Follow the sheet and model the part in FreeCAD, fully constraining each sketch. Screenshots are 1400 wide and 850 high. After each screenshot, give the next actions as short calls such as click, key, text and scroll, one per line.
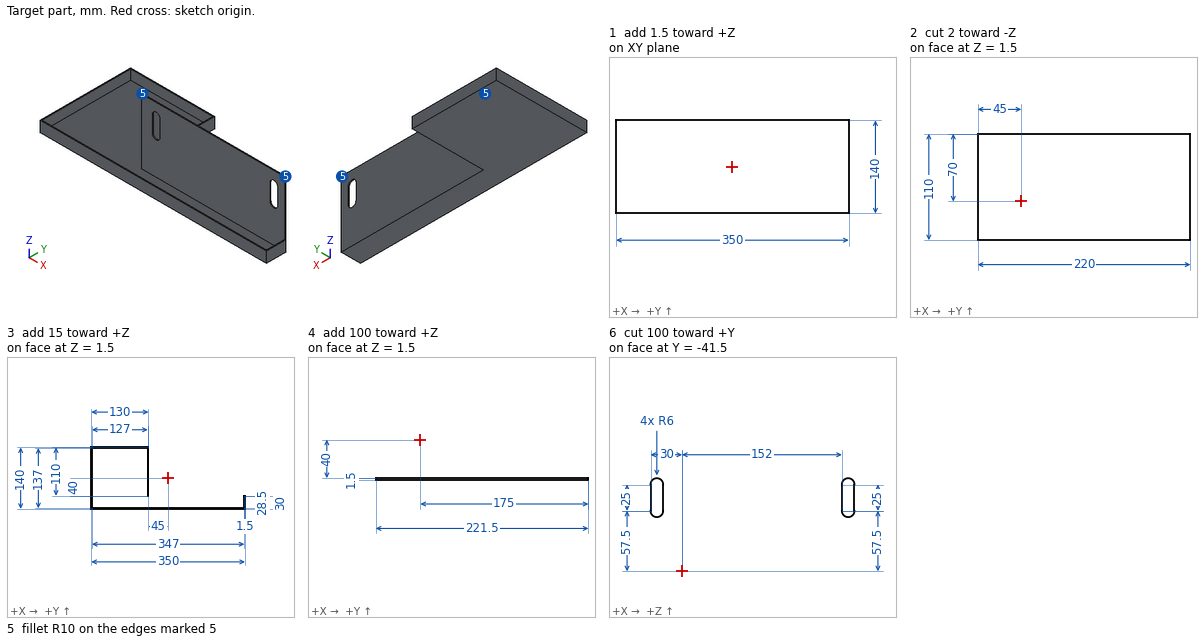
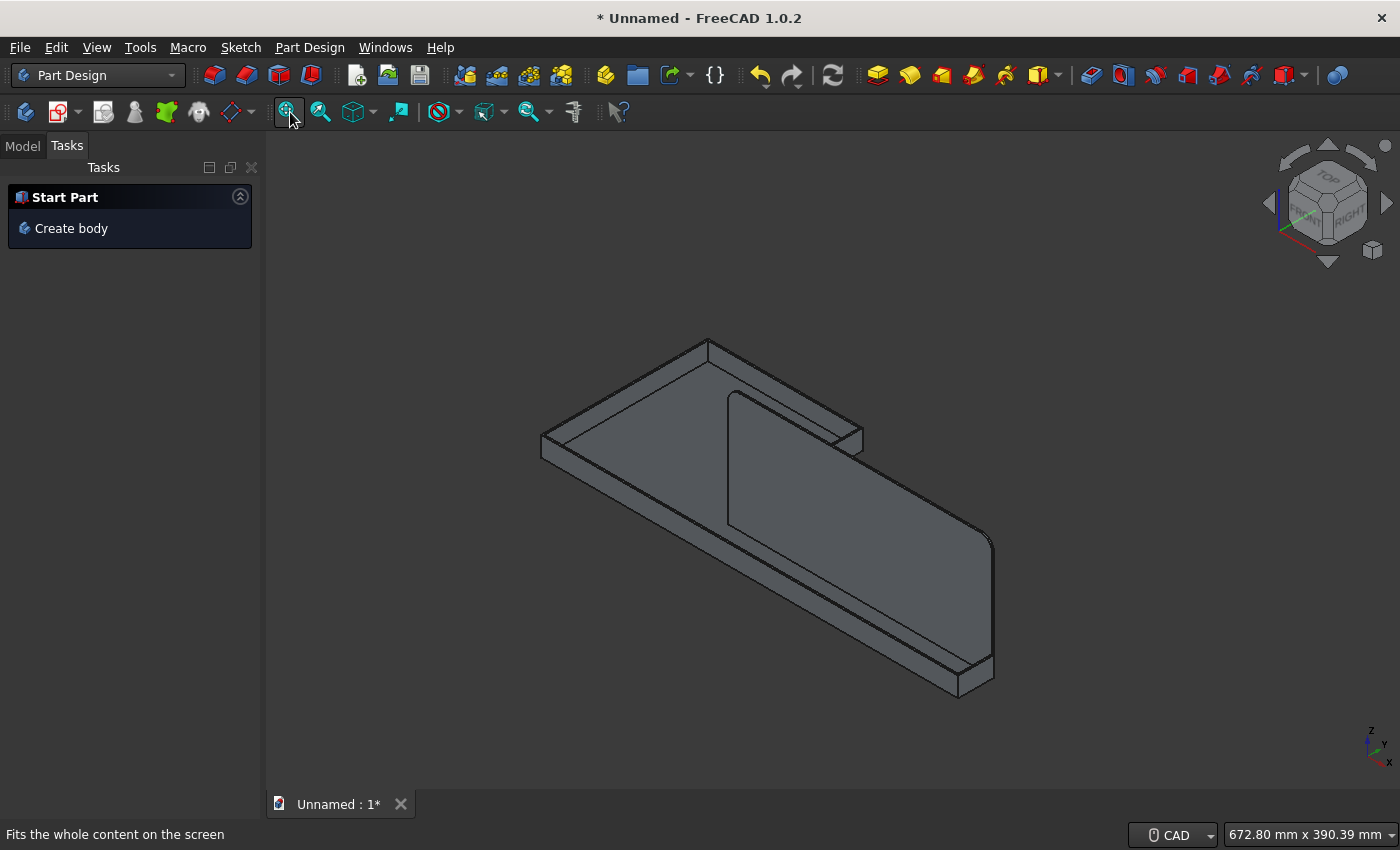
click(898, 553)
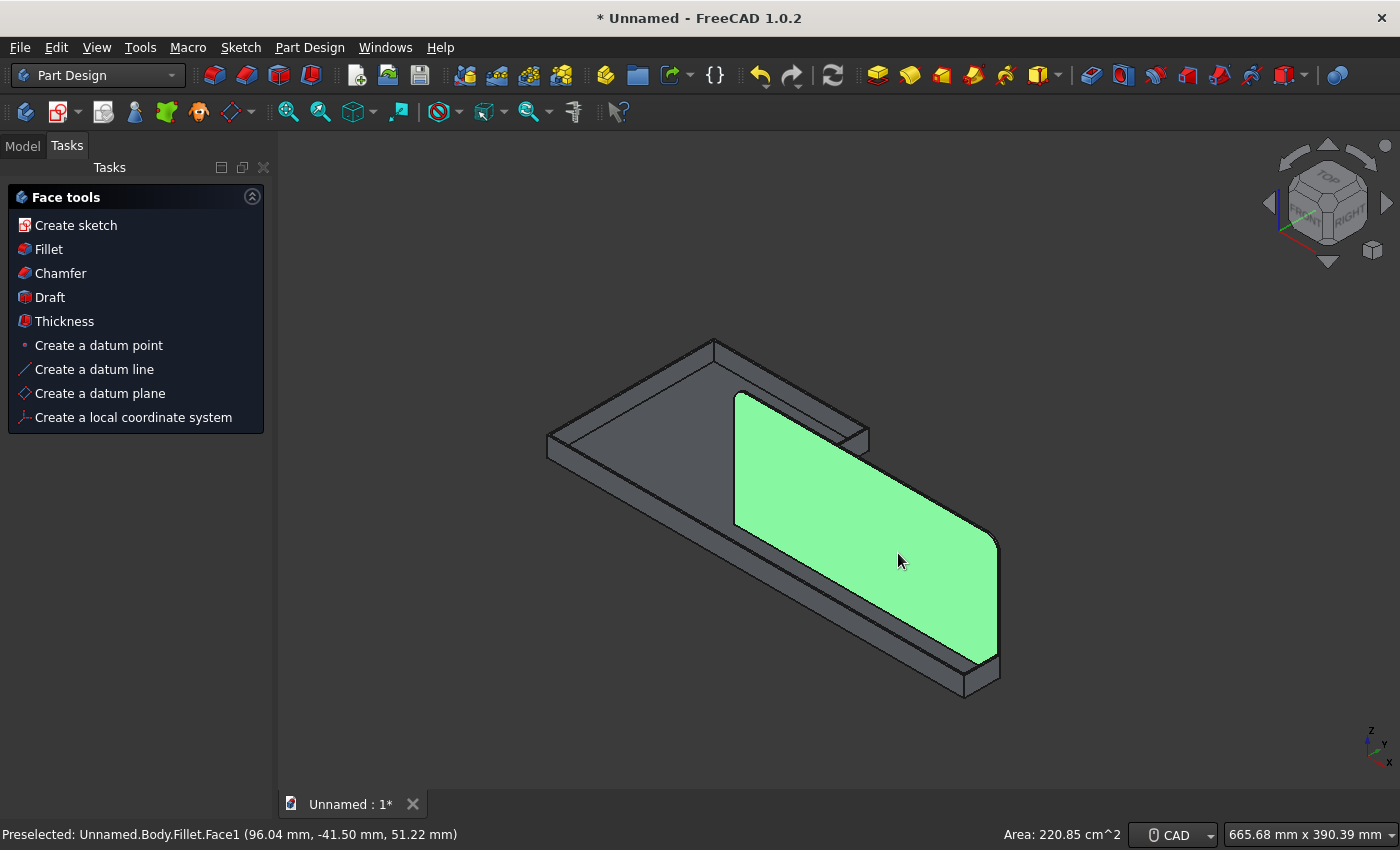
click(58, 112)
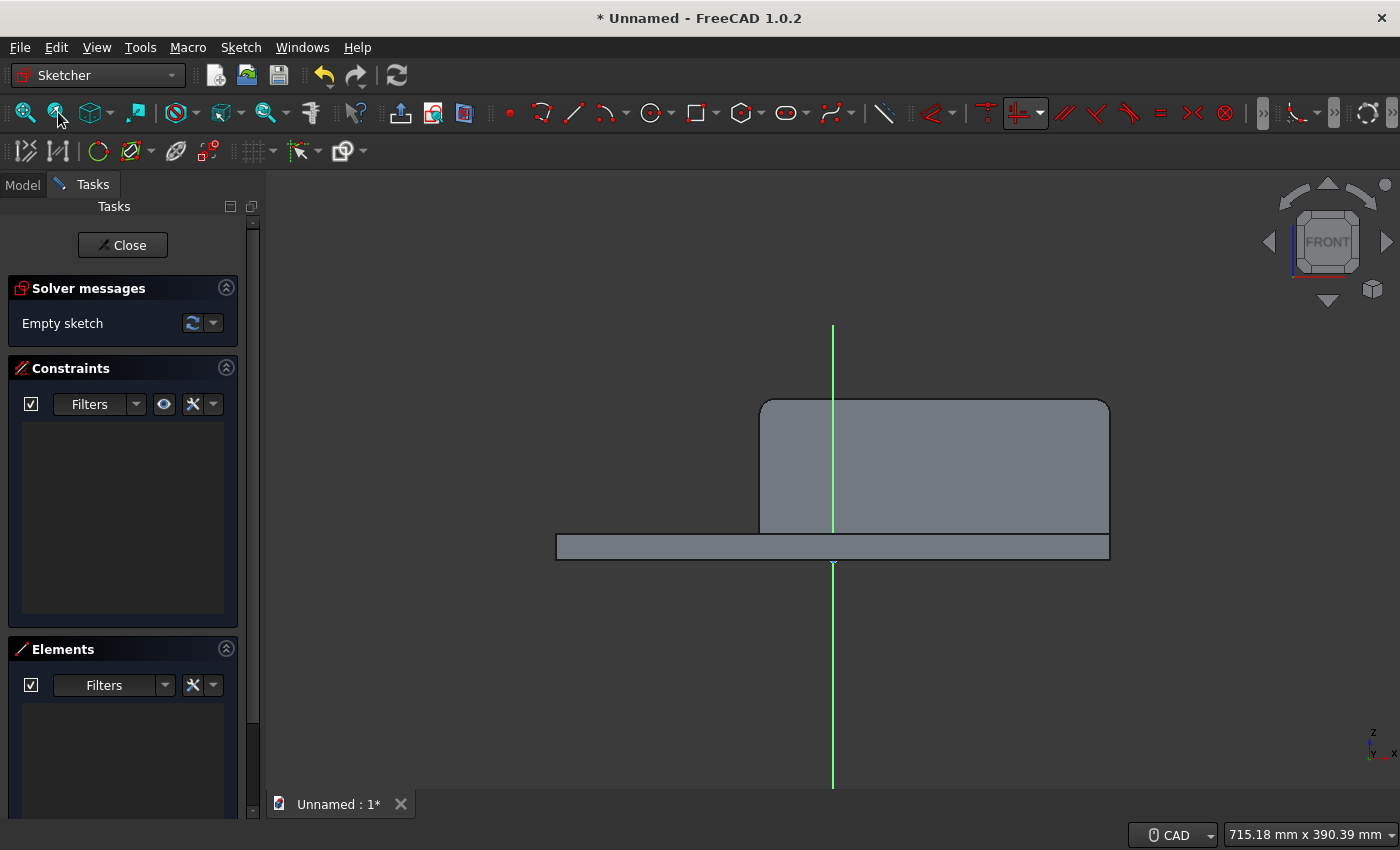
click(466, 114)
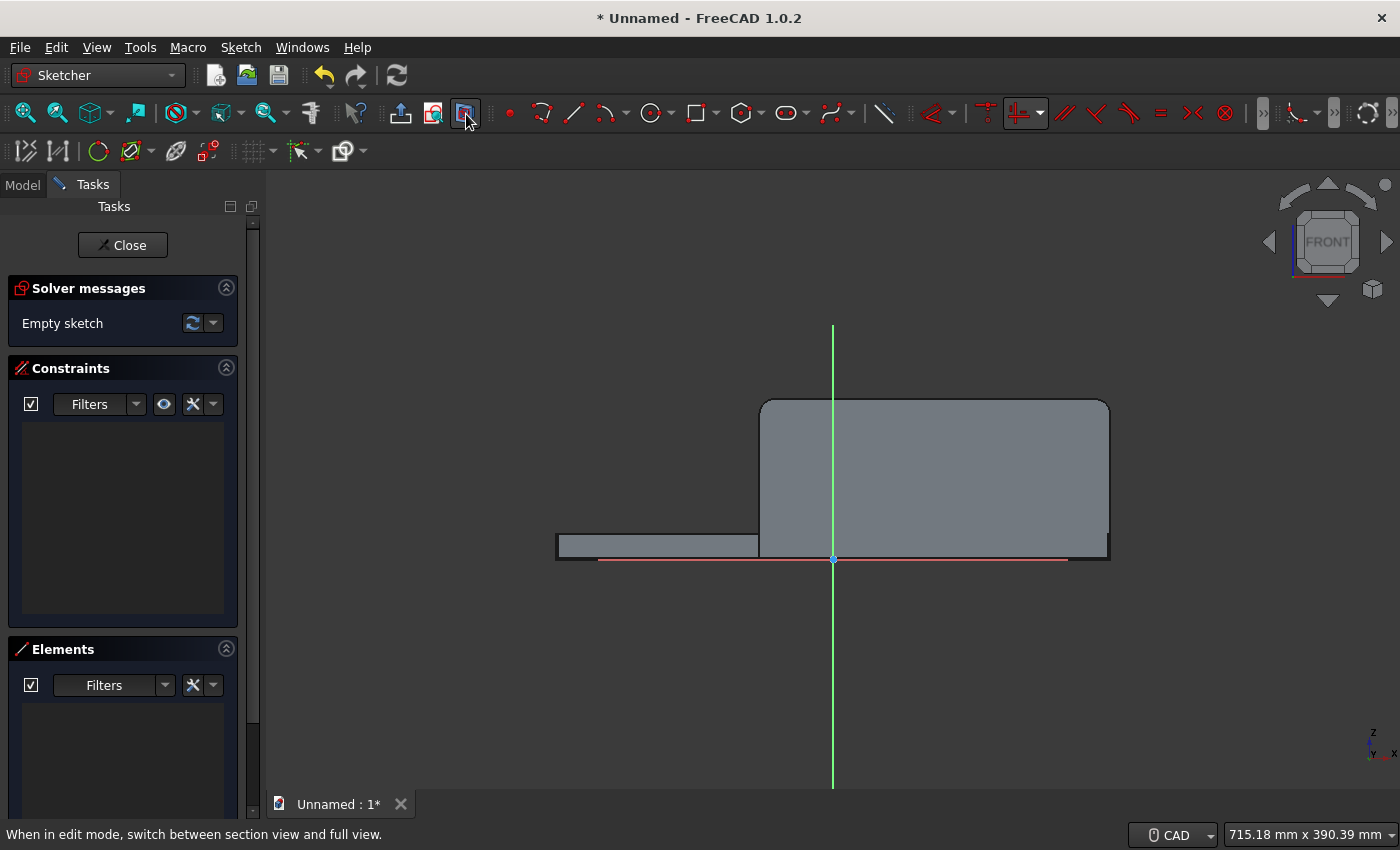
scroll(1082, 498, up, 4)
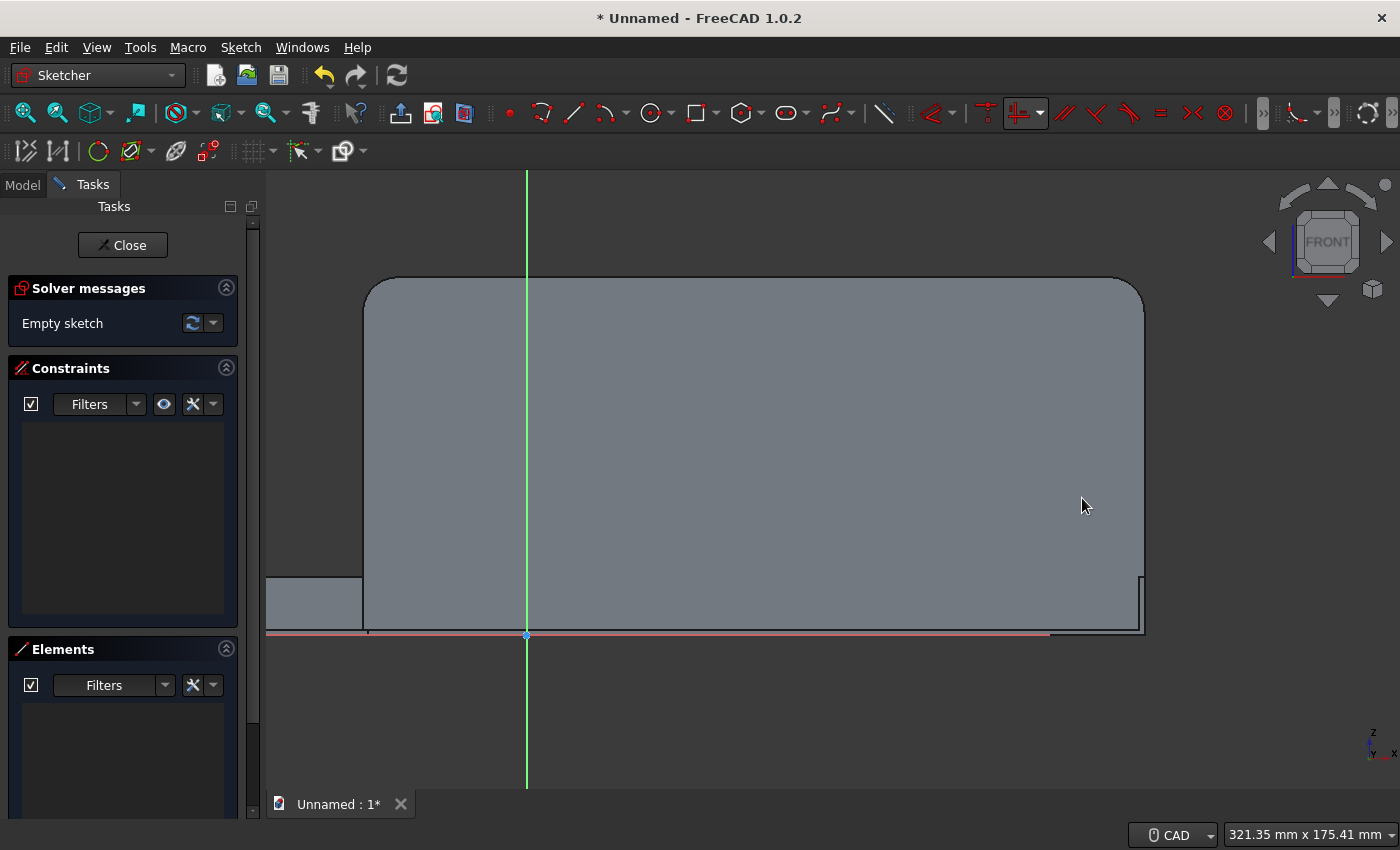
click(786, 114)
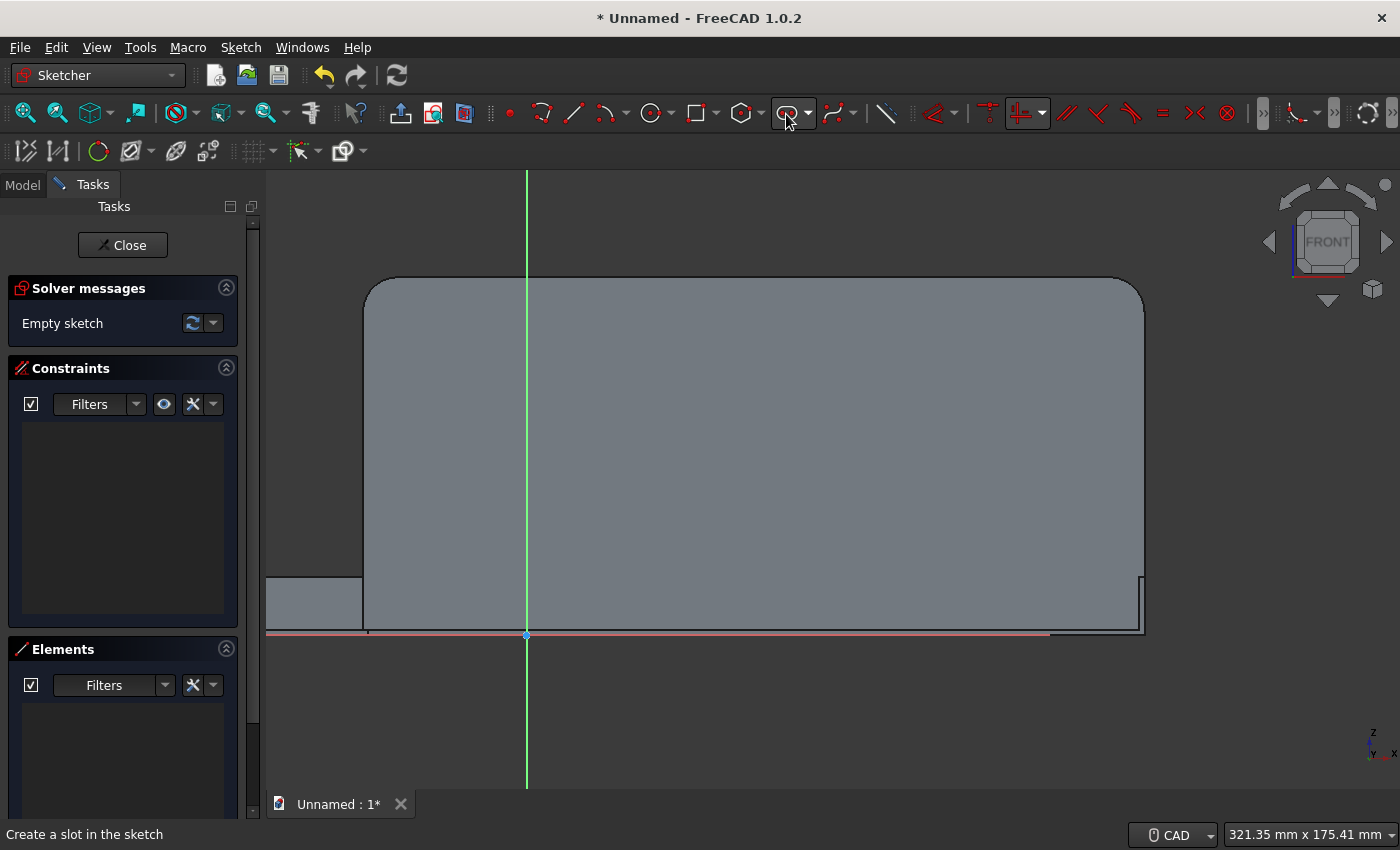
click(442, 432)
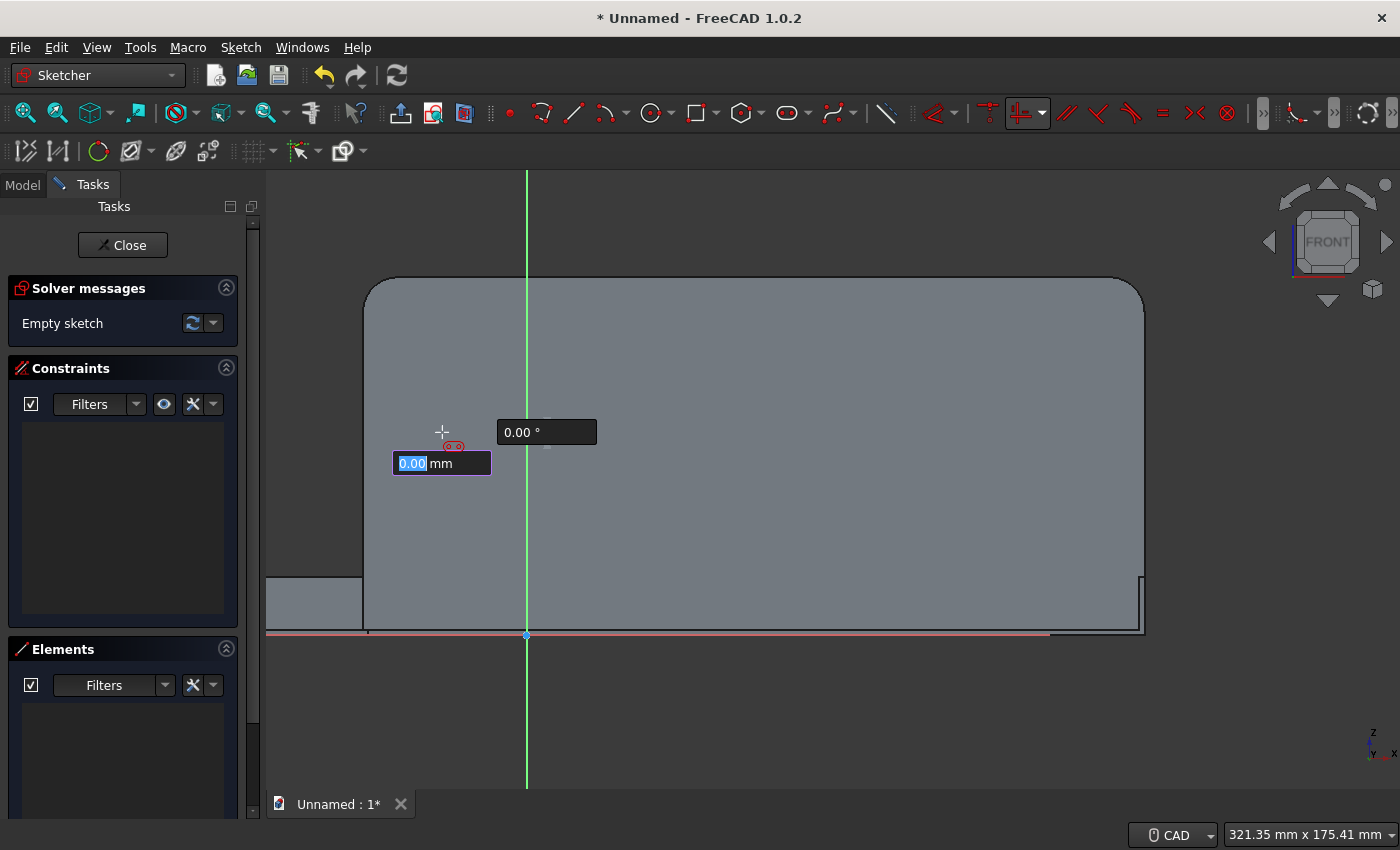
click(442, 344)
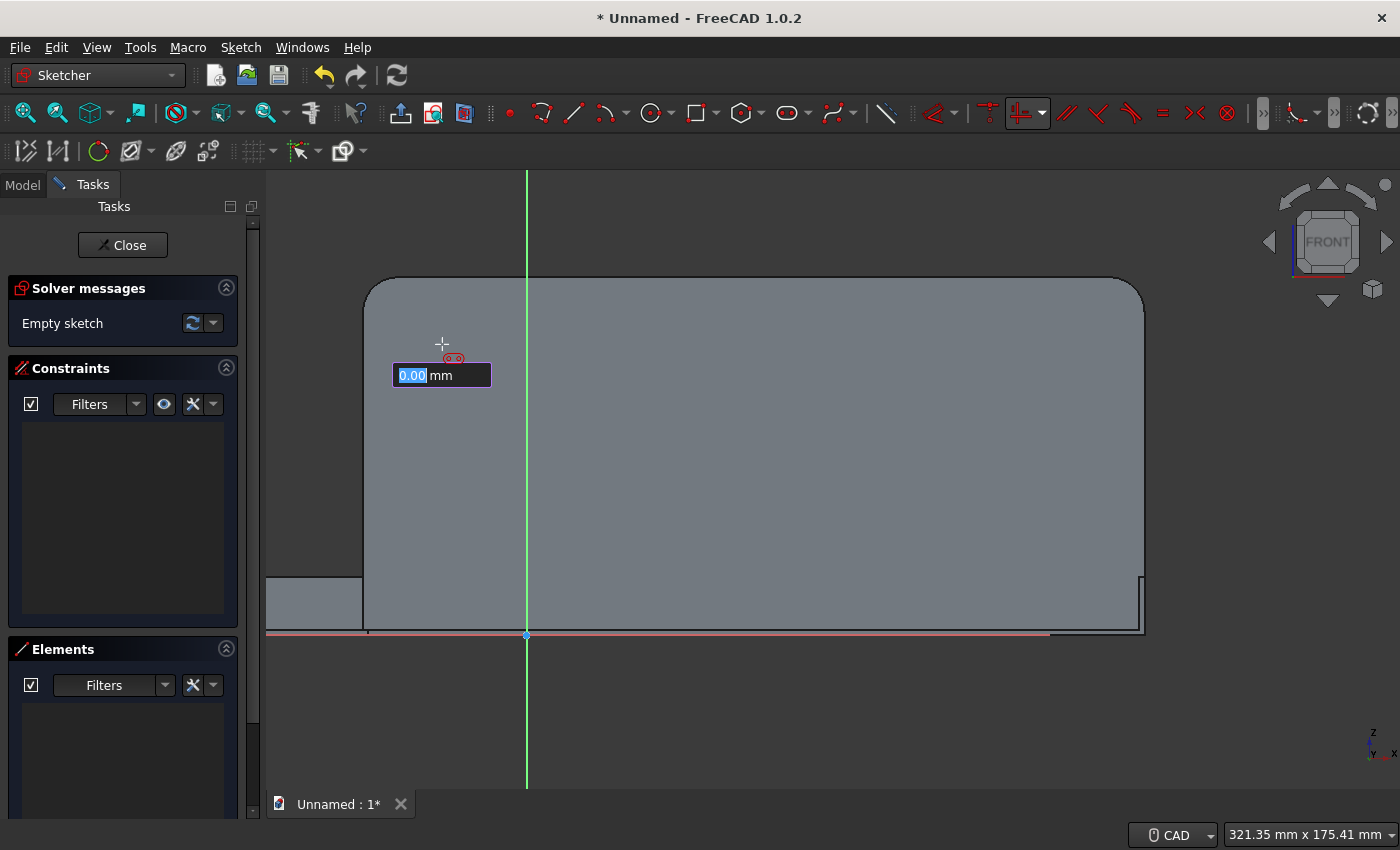
click(463, 388)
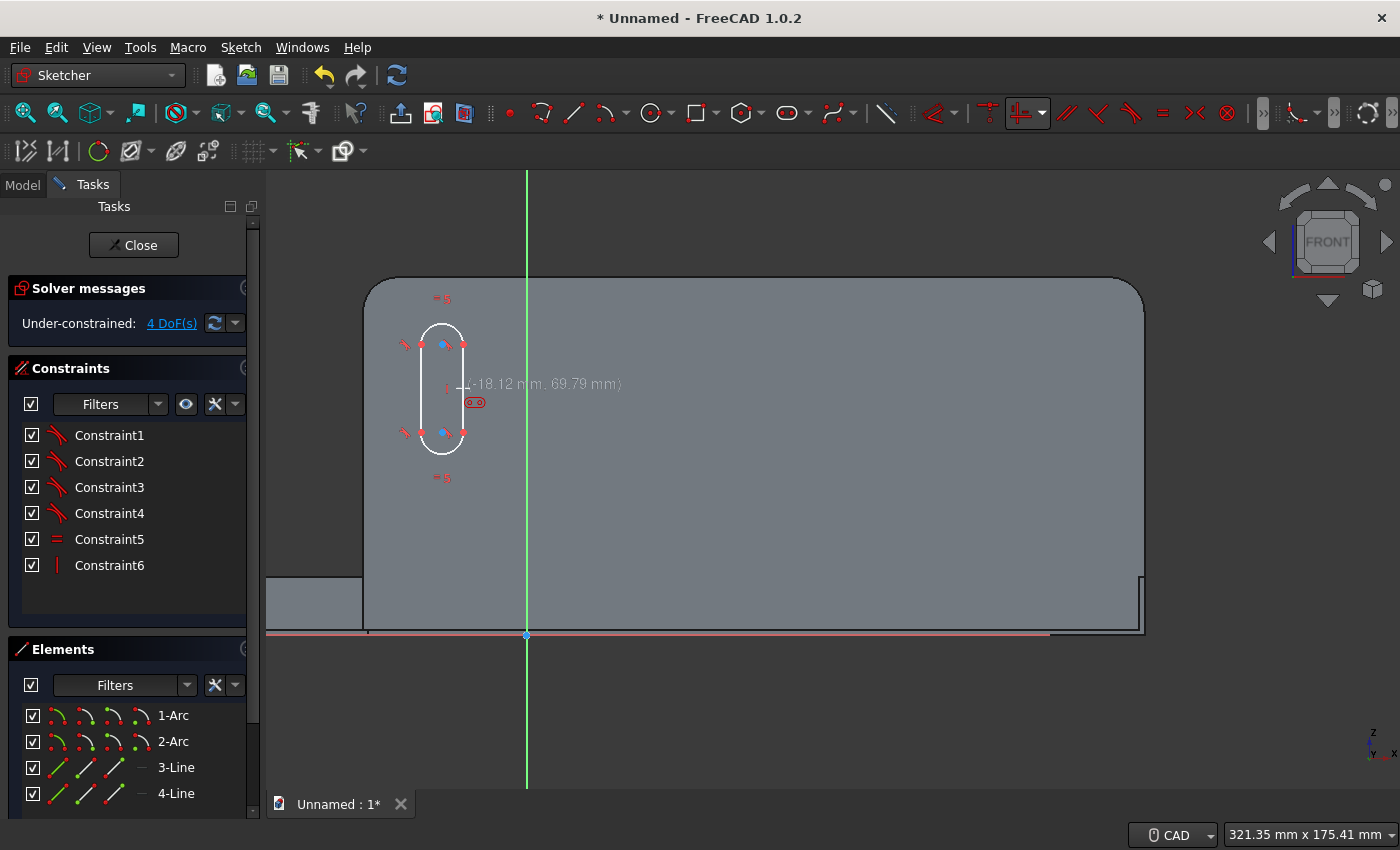
click(1085, 432)